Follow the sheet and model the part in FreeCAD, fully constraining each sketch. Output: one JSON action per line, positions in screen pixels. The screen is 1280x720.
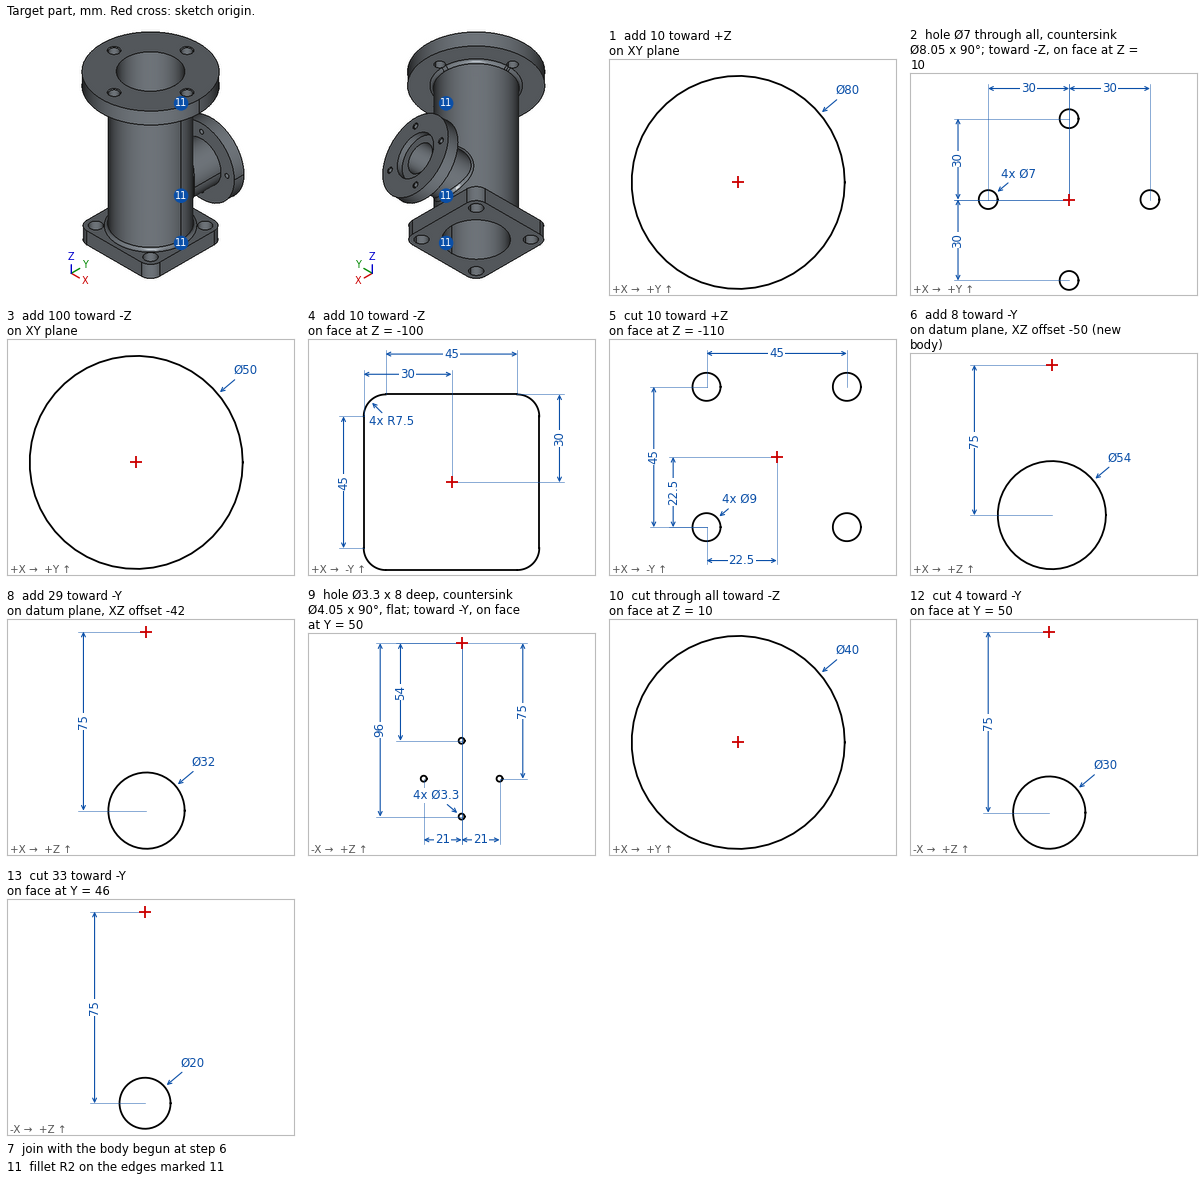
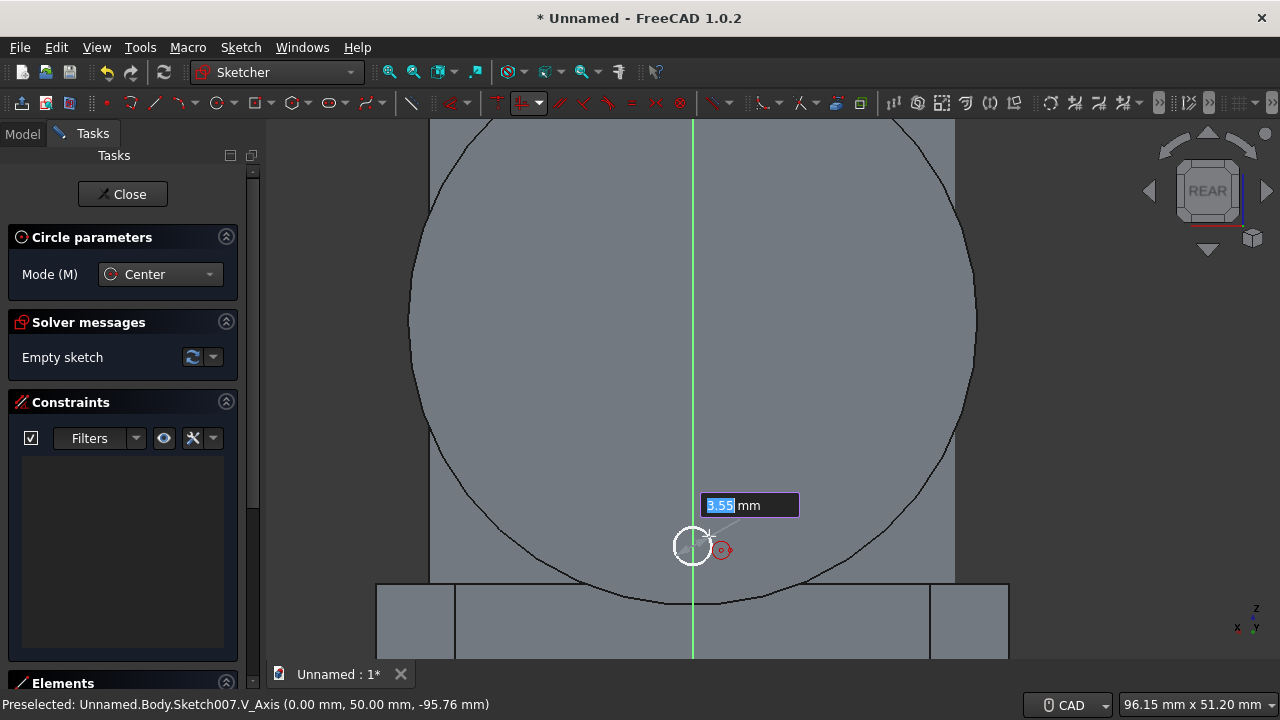
{"action": "type", "text": "3.3"}
{"action": "key", "text": "Return"}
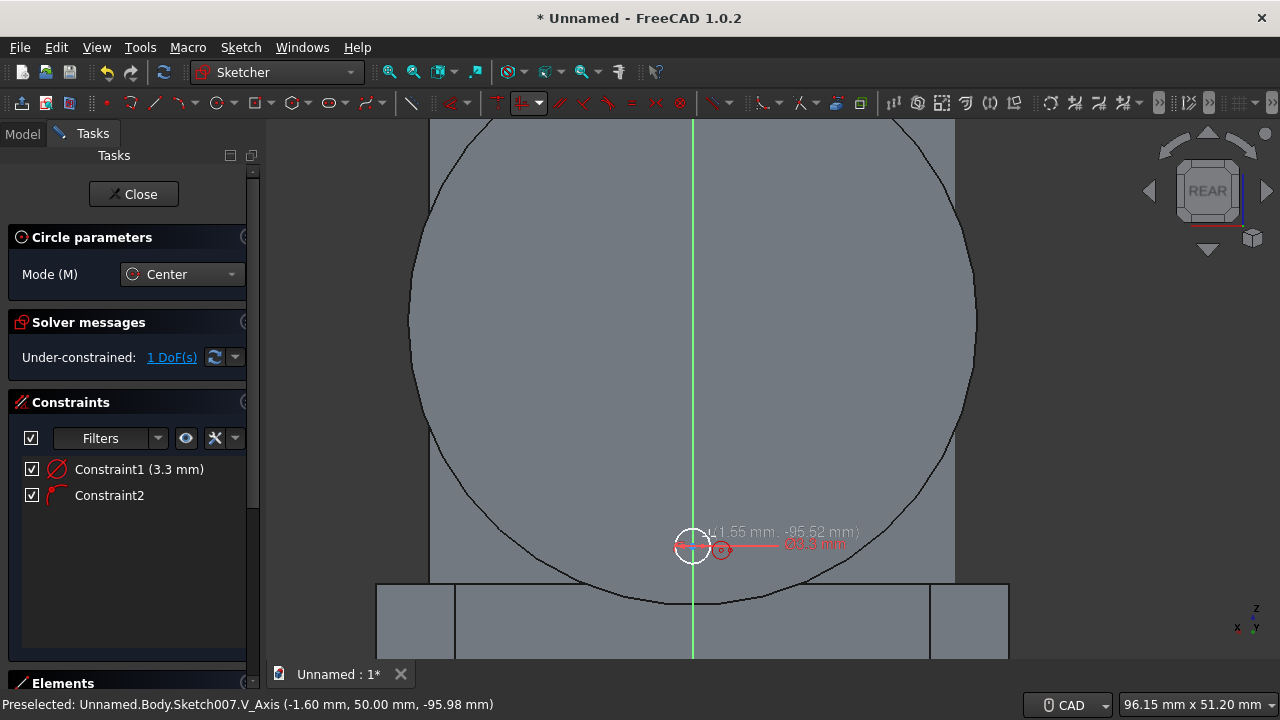
{"action": "scroll", "coordinate": [914, 321], "scroll_direction": "up", "scroll_amount": 2}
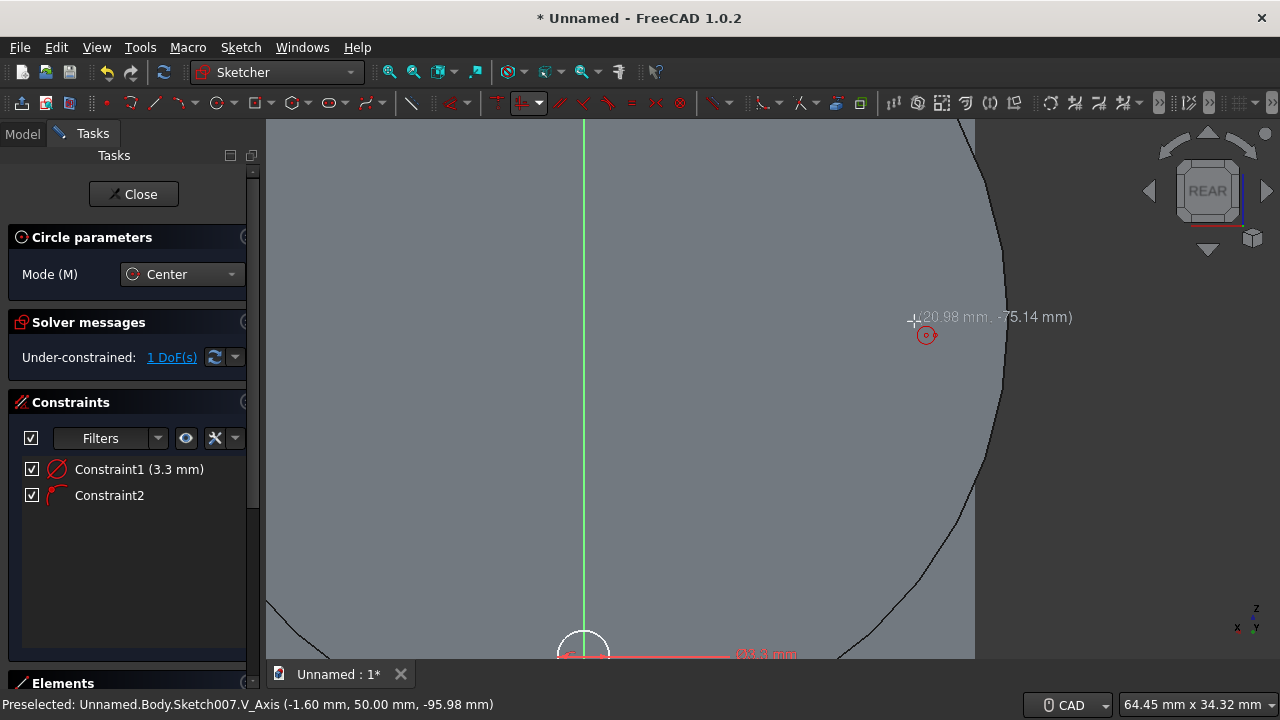
{"action": "scroll", "coordinate": [735, 511], "scroll_direction": "down", "scroll_amount": 8}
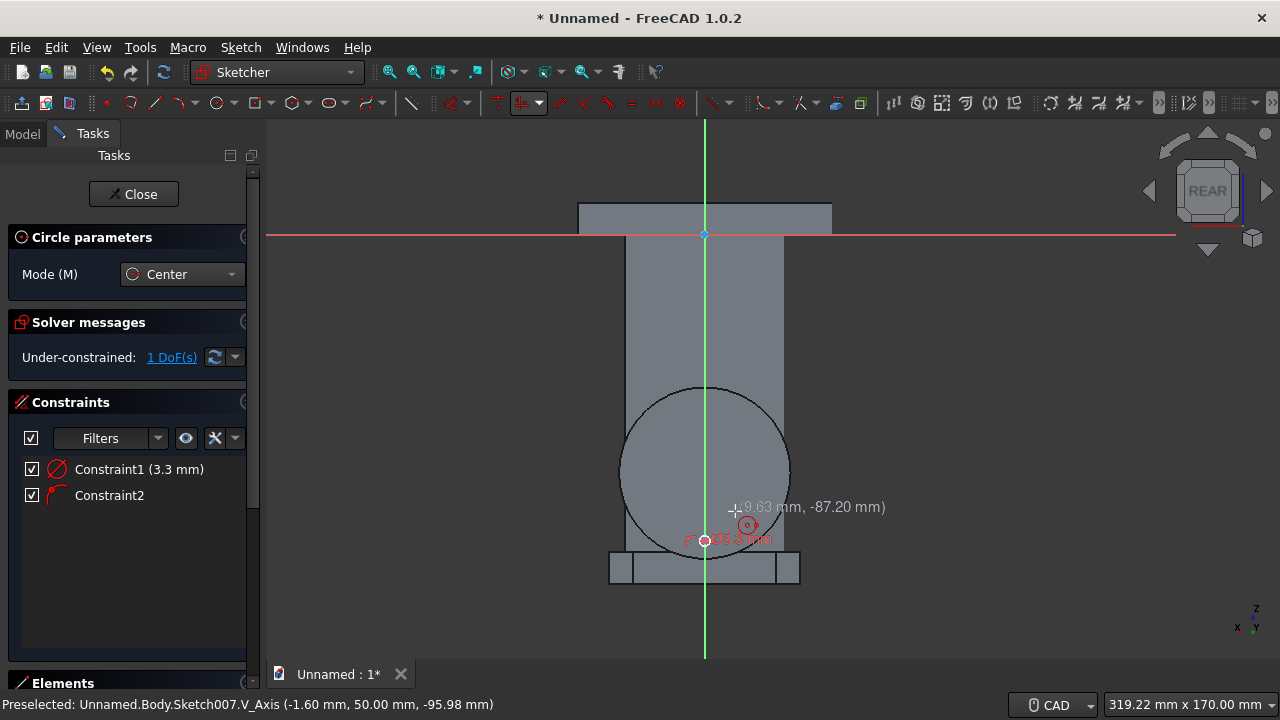
{"action": "left_click", "coordinate": [771, 473]}
{"action": "mouse_move", "coordinate": [775, 469]}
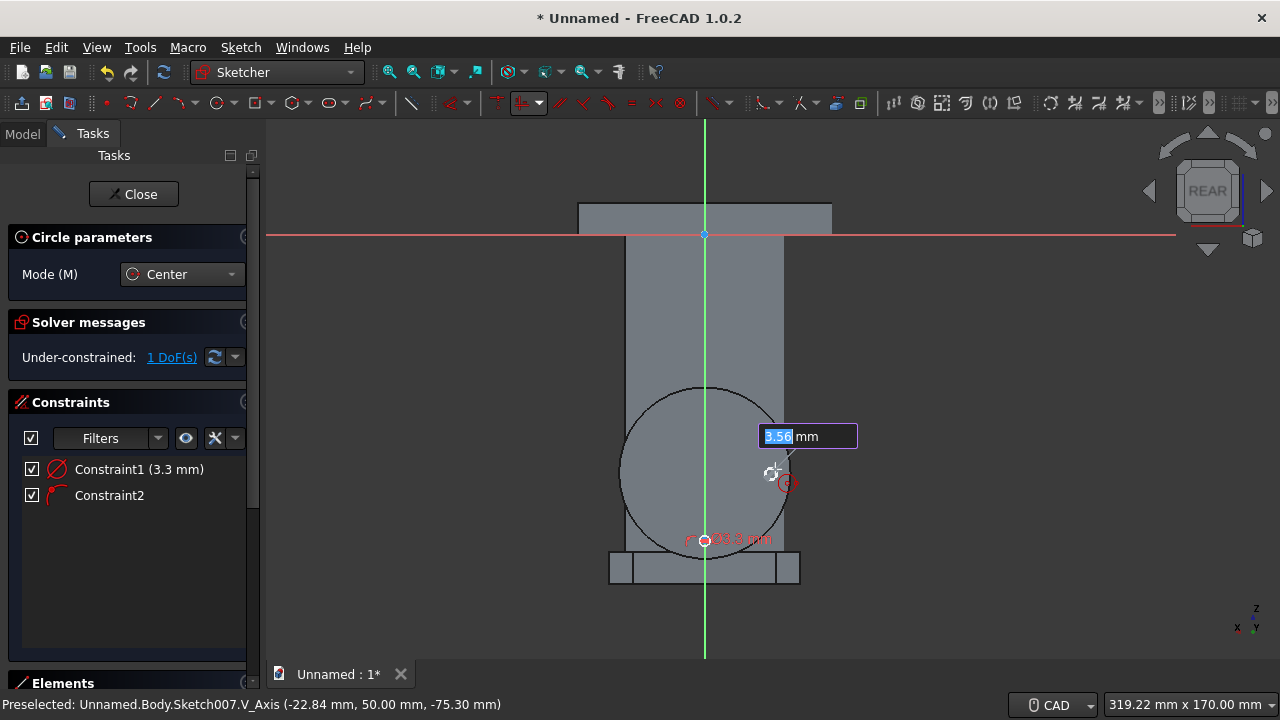
{"action": "type", "text": "3.3"}
{"action": "key", "text": "Return"}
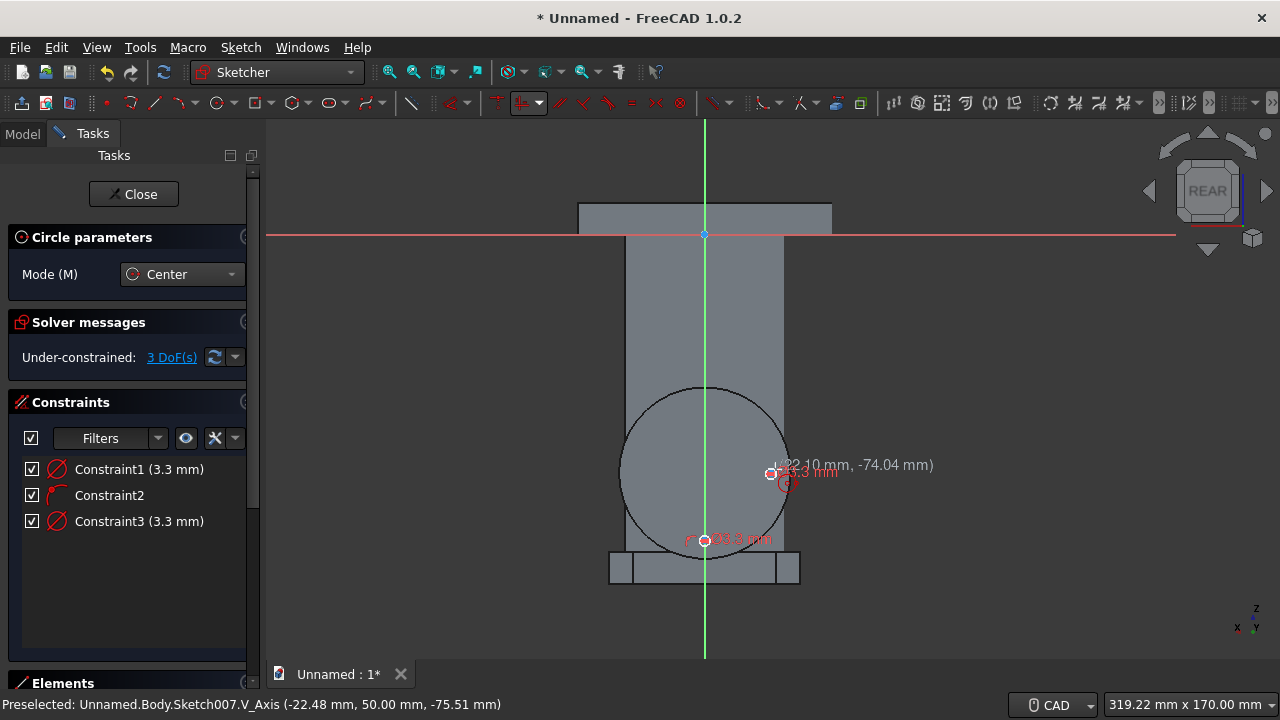
{"action": "scroll", "coordinate": [705, 406], "scroll_direction": "up", "scroll_amount": 8}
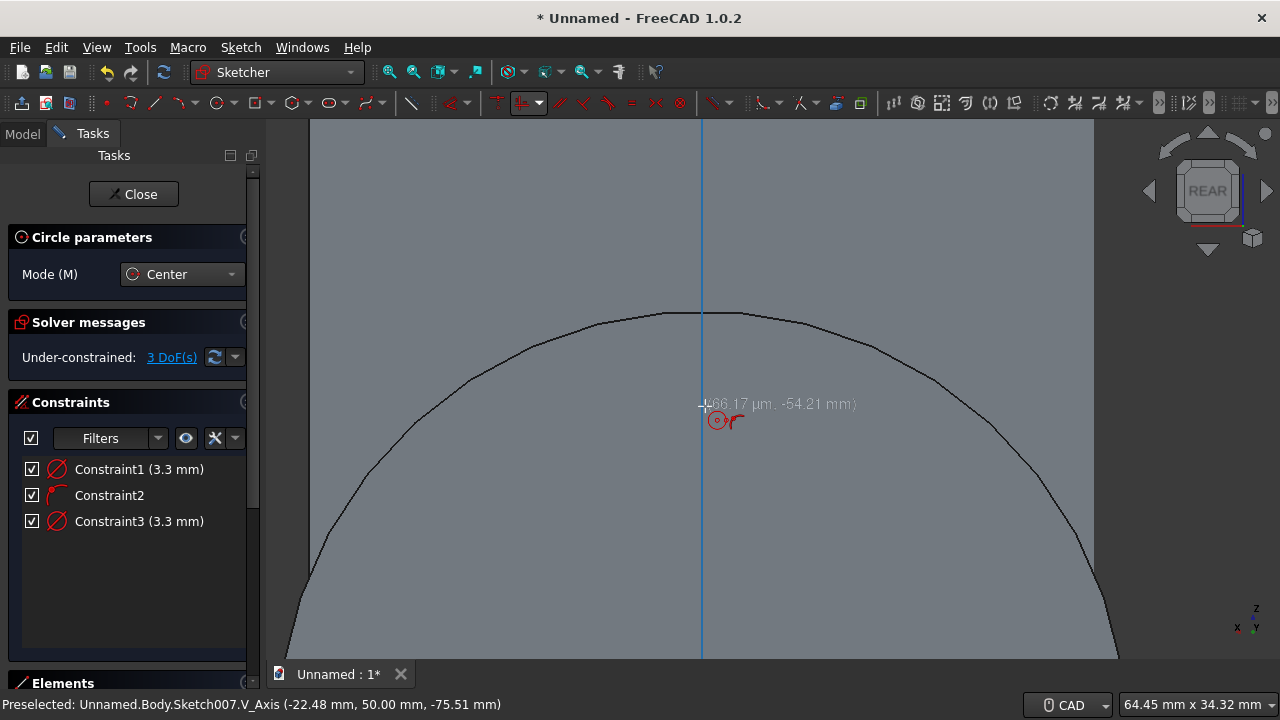
{"action": "scroll", "coordinate": [705, 405], "scroll_direction": "down", "scroll_amount": 8}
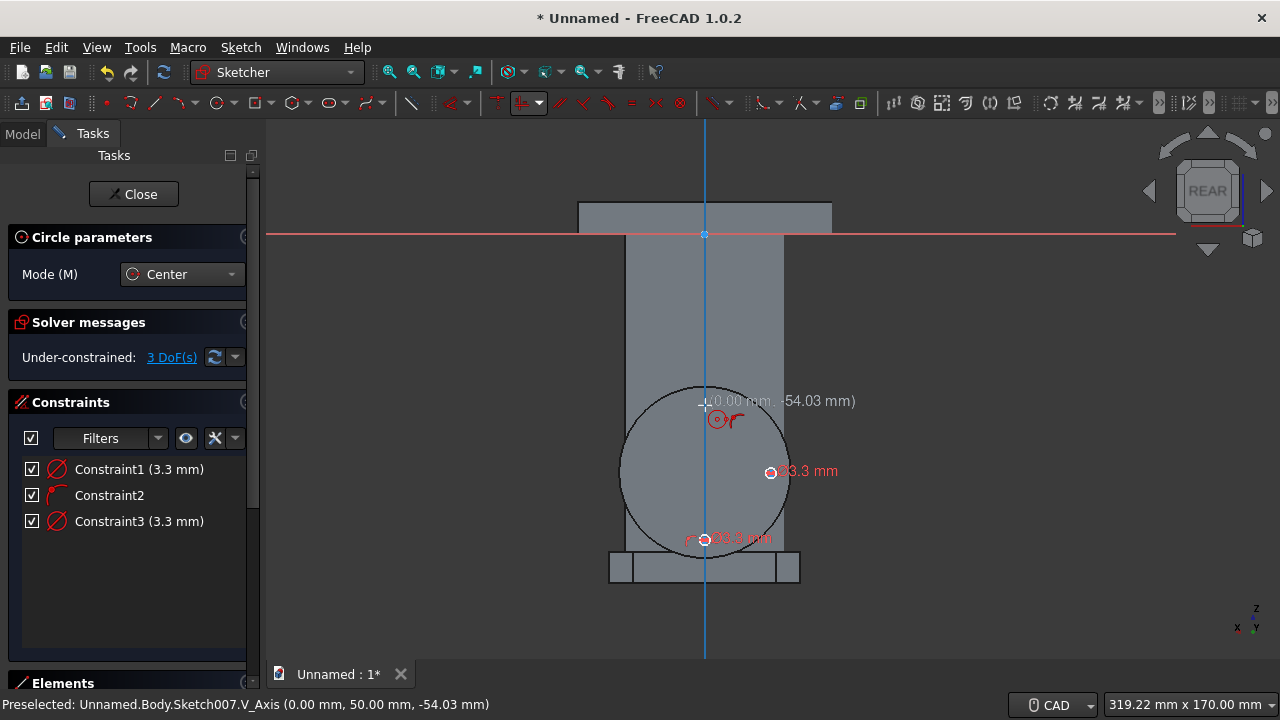
{"action": "left_click", "coordinate": [705, 406]}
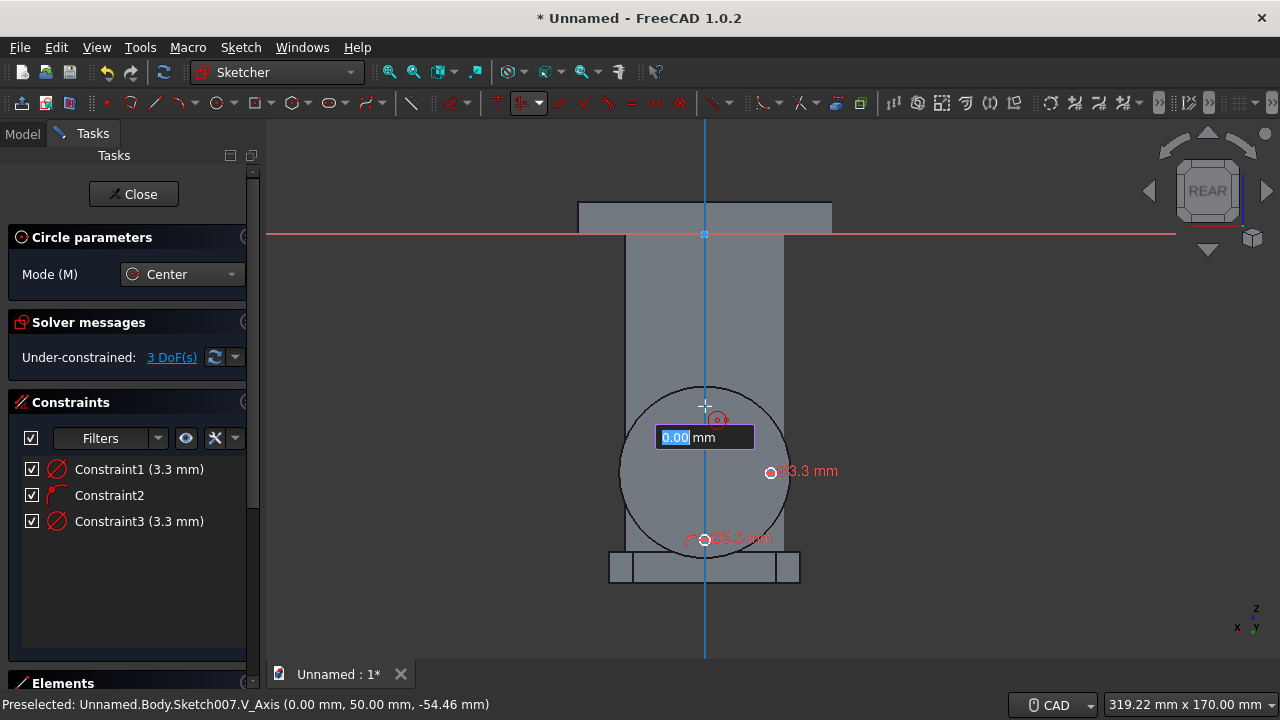
{"action": "scroll", "coordinate": [710, 404], "scroll_direction": "up", "scroll_amount": 6}
{"action": "mouse_move", "coordinate": [708, 402]}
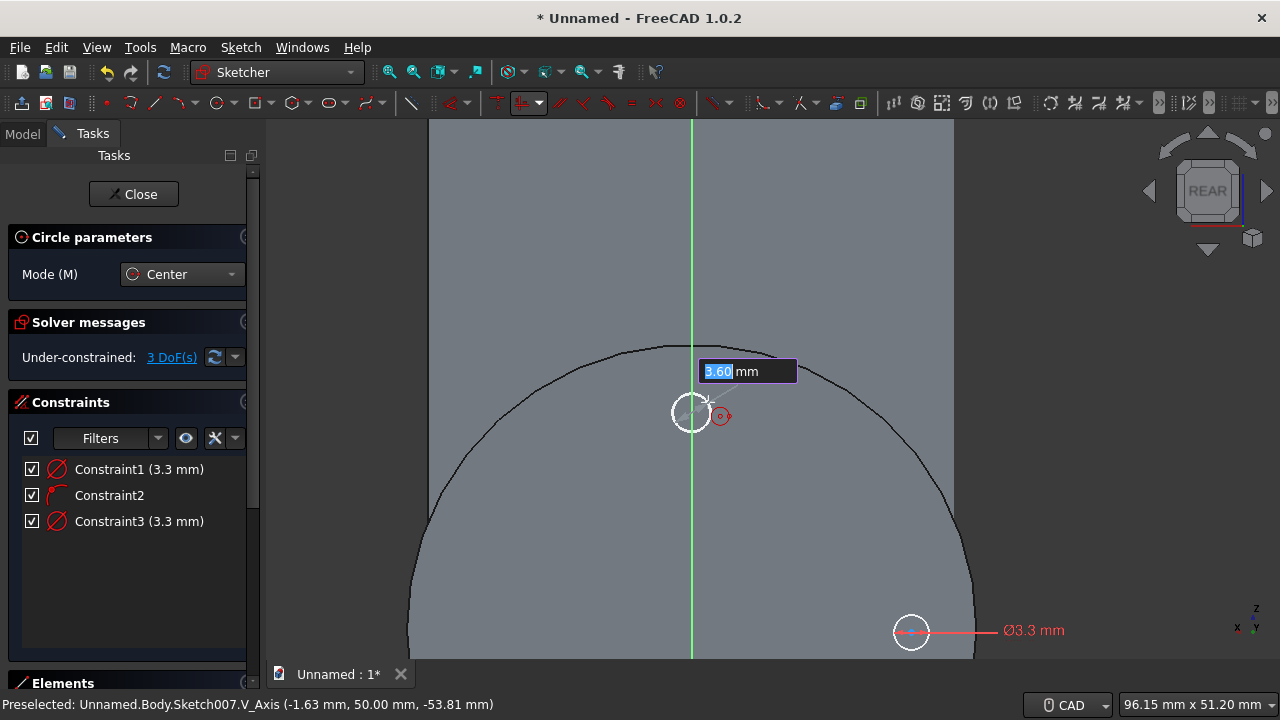
{"action": "type", "text": "3.3"}
{"action": "key", "text": "Return"}